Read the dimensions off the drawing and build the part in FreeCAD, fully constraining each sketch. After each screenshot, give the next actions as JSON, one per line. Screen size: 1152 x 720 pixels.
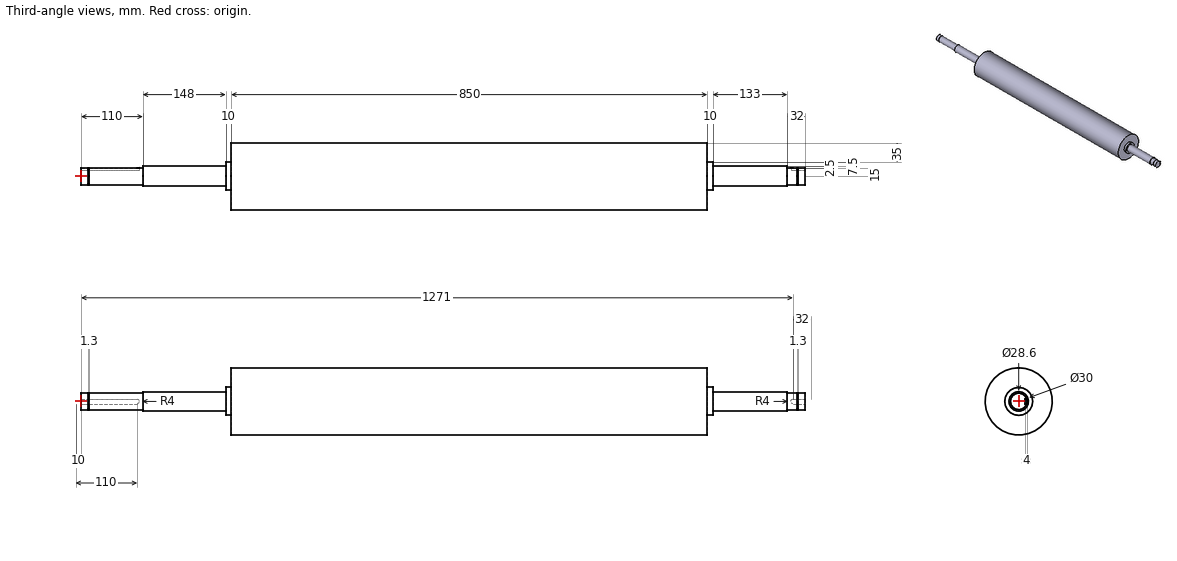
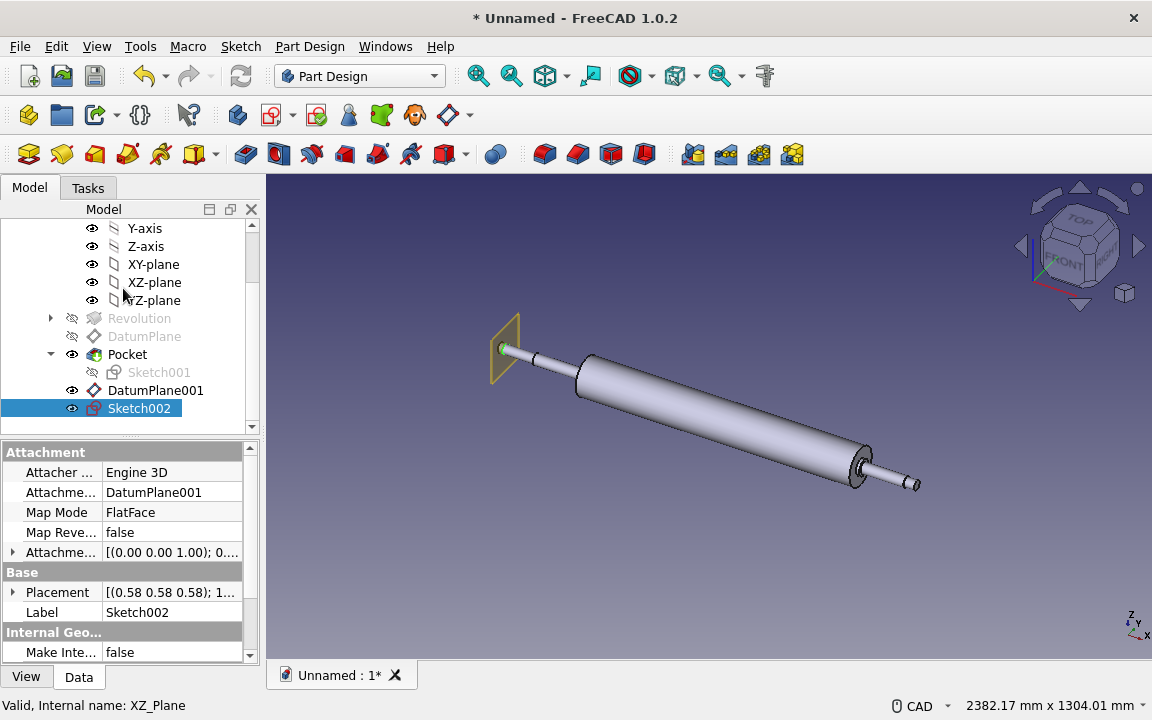
{"action": "left_click", "coordinate": [246, 154]}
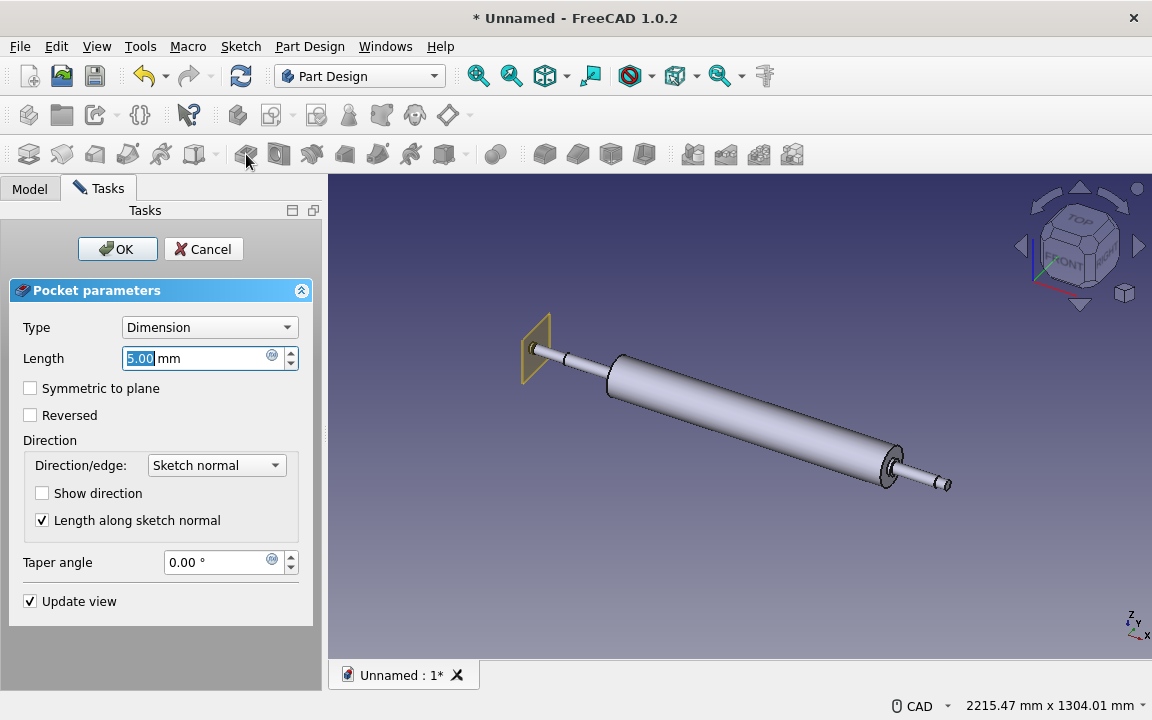
{"action": "type", "text": "1.3"}
{"action": "key", "text": "Tab"}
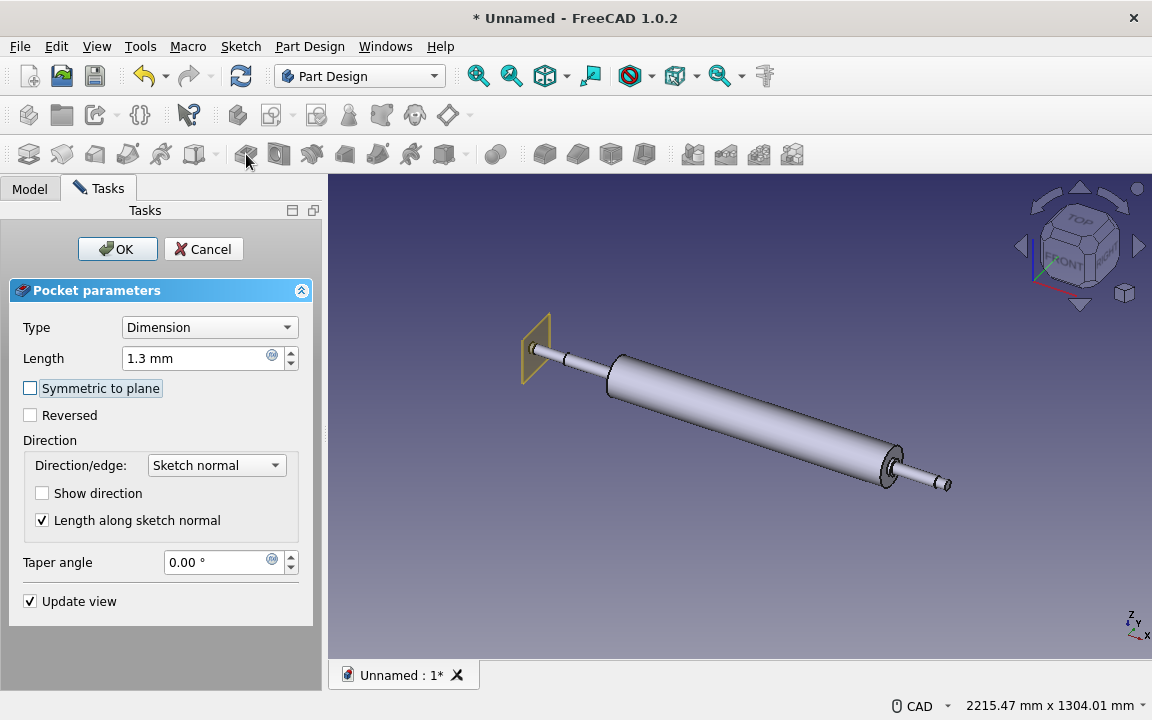
{"action": "left_click", "coordinate": [118, 249]}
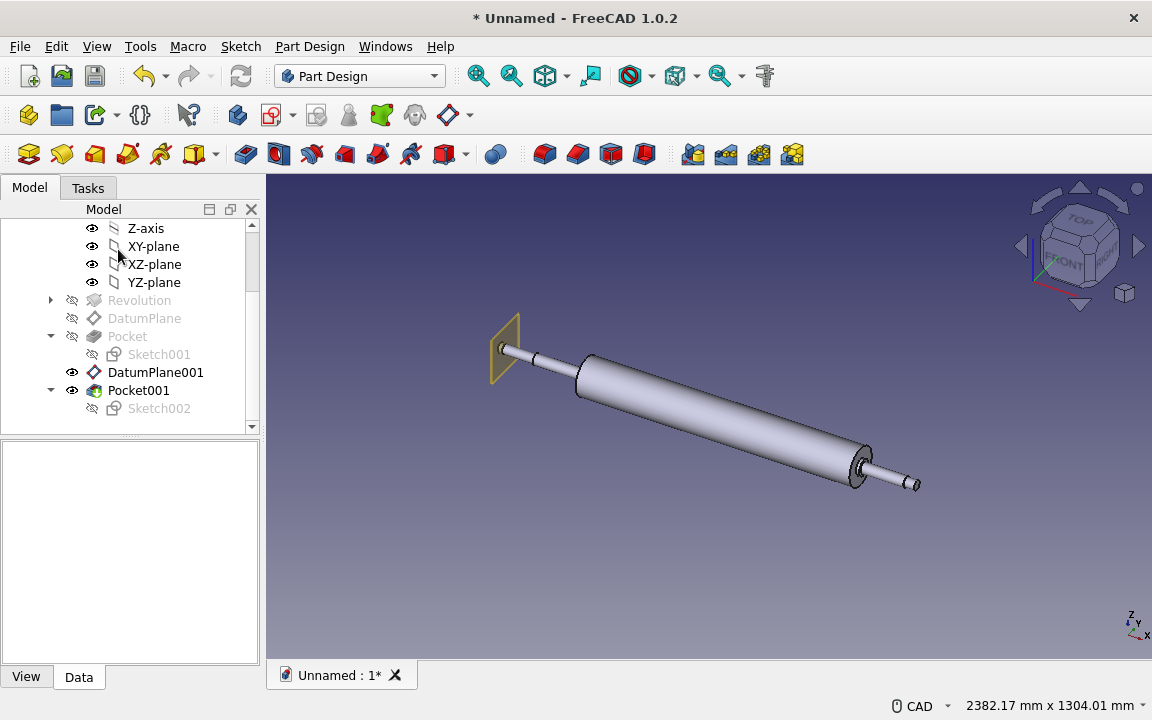
{"action": "left_click", "coordinate": [117, 372]}
{"action": "key", "text": "space"}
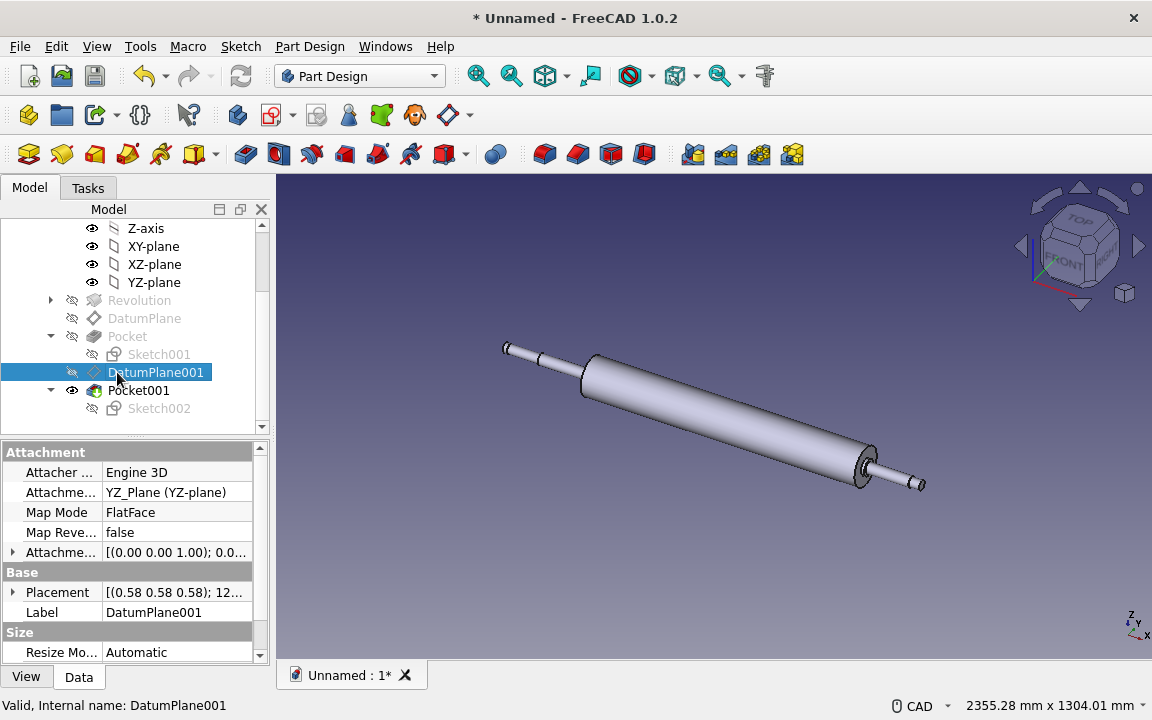
{"action": "scroll", "coordinate": [161, 314], "scroll_direction": "down", "scroll_amount": 3}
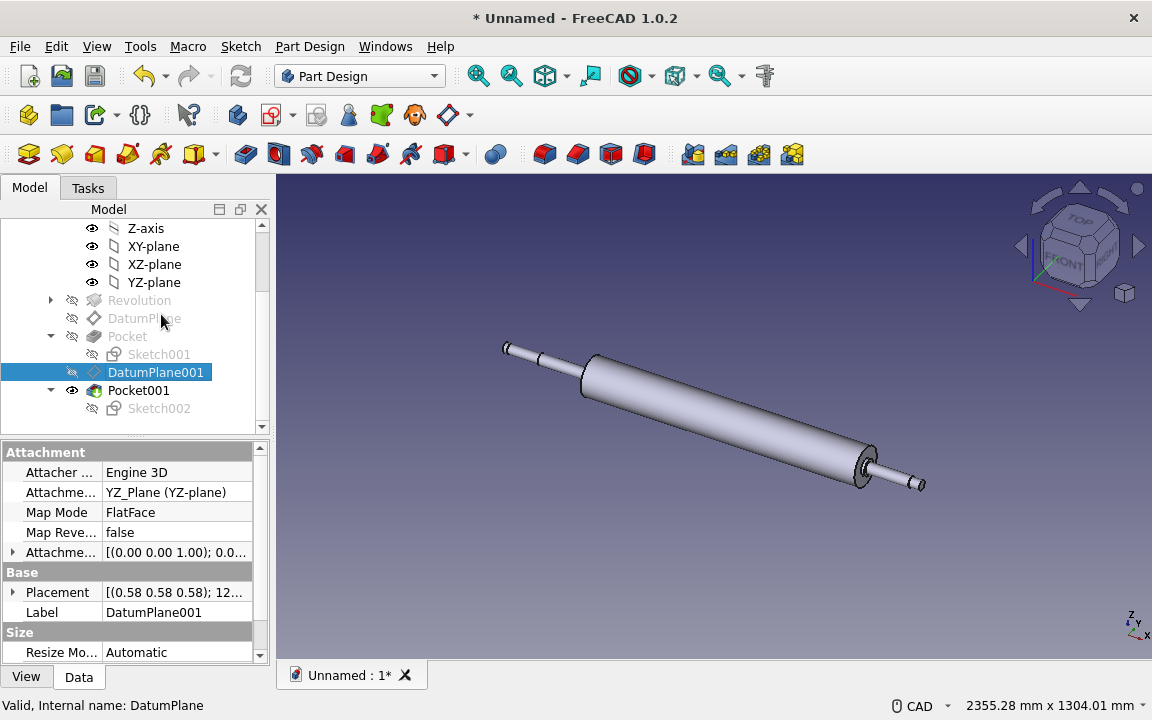
{"action": "scroll", "coordinate": [161, 314], "scroll_direction": "up", "scroll_amount": 15}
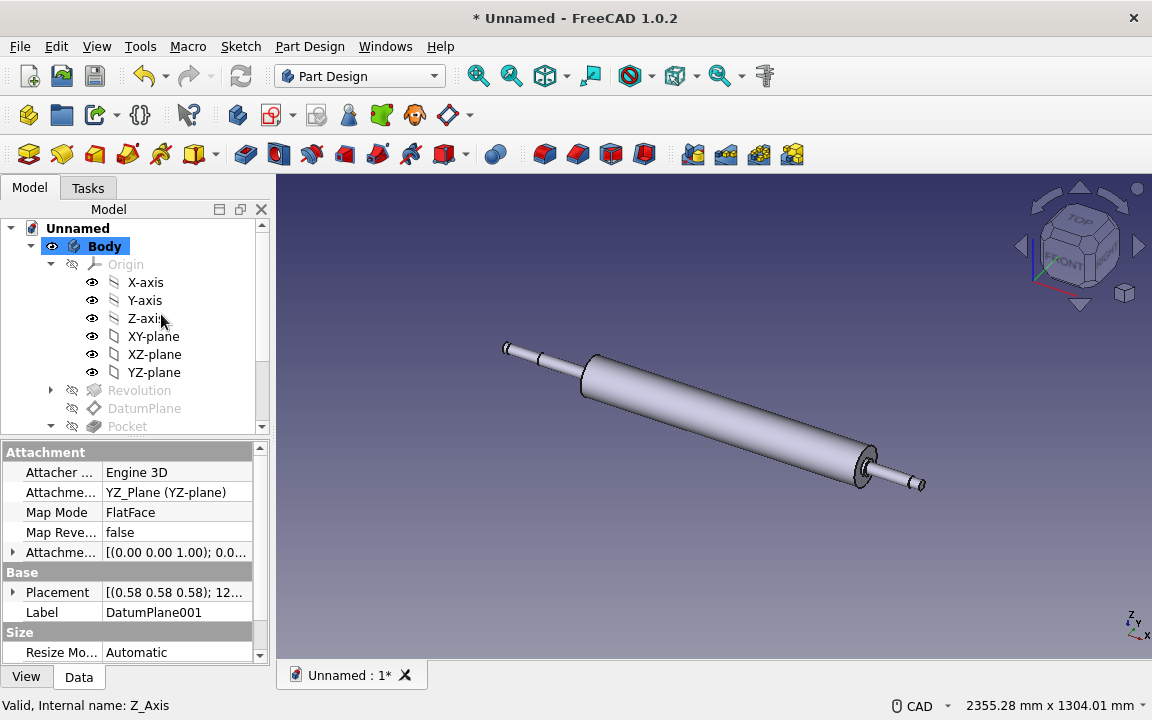
{"action": "left_click", "coordinate": [137, 354]}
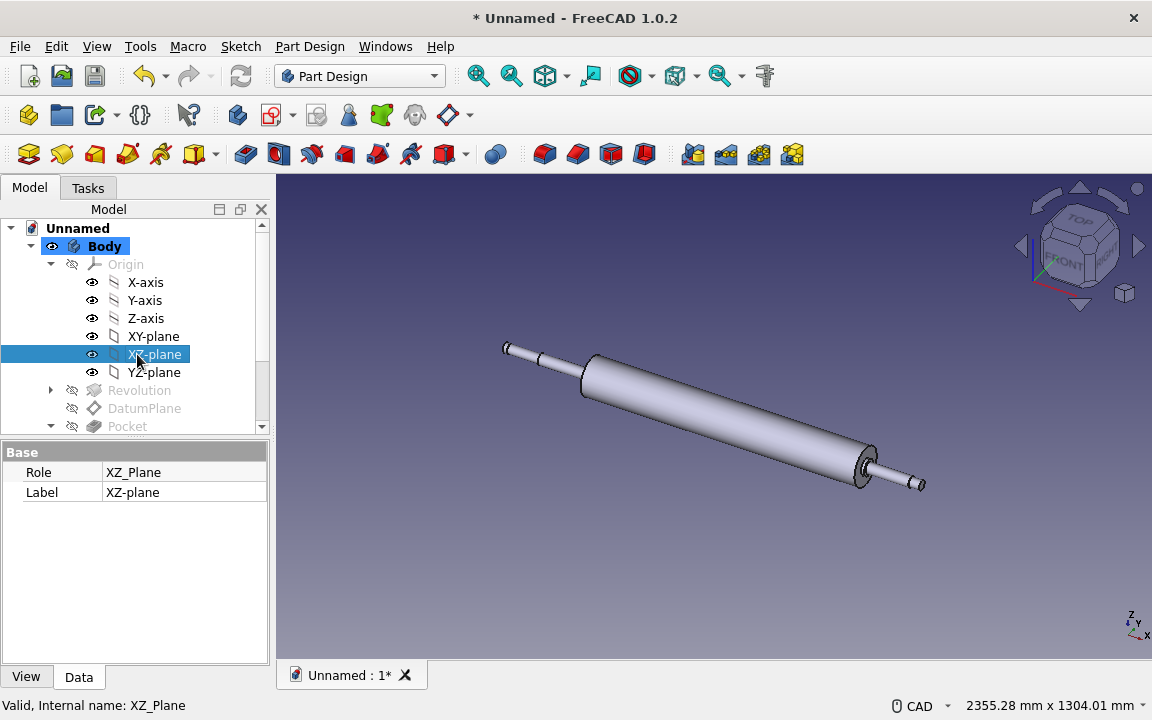
{"action": "left_click", "coordinate": [448, 116]}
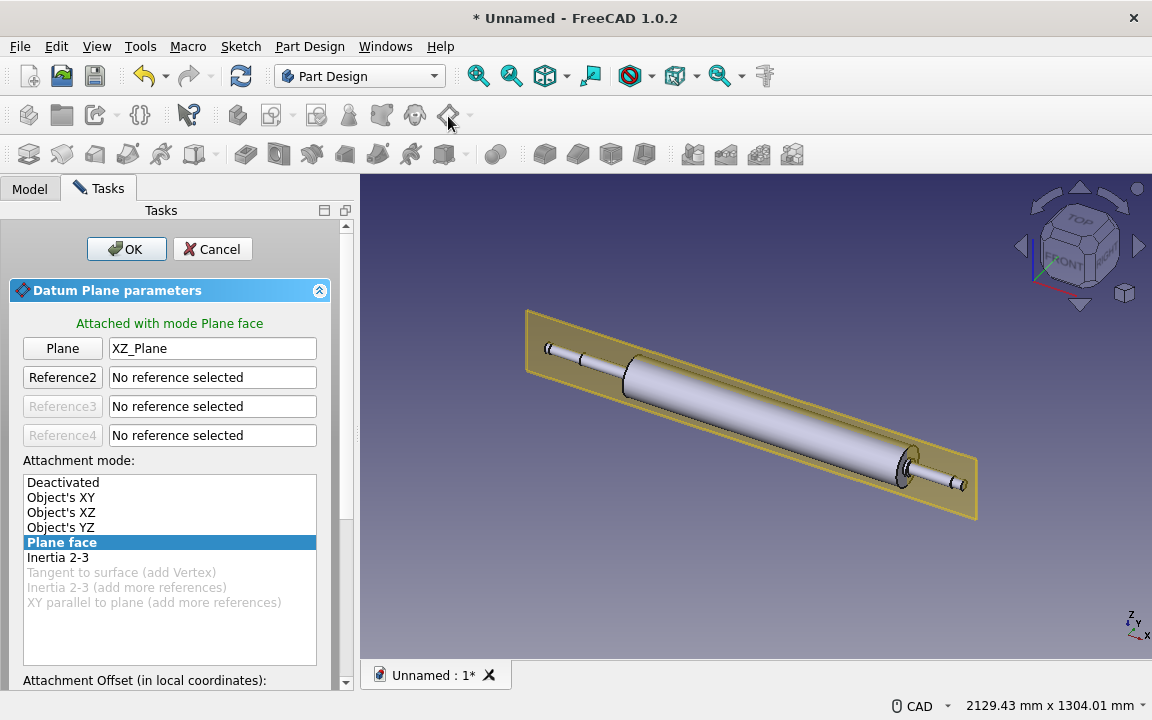
{"action": "scroll", "coordinate": [346, 455], "scroll_direction": "down", "scroll_amount": 3}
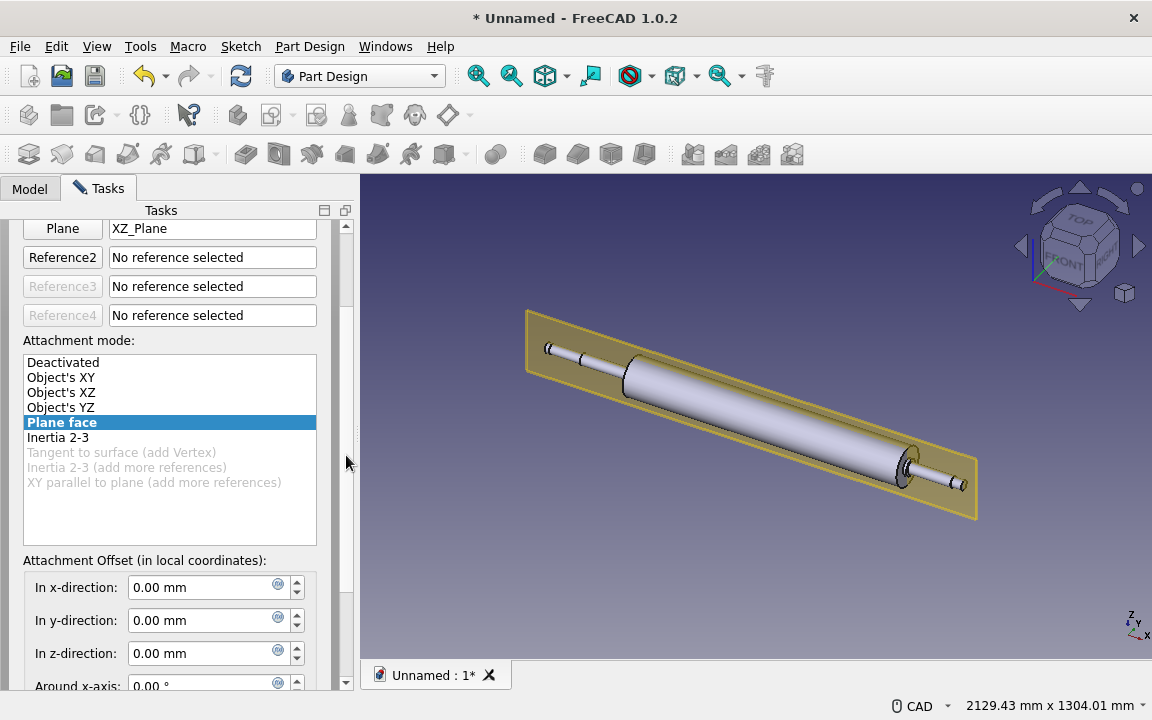
{"action": "triple_click", "coordinate": [210, 594]}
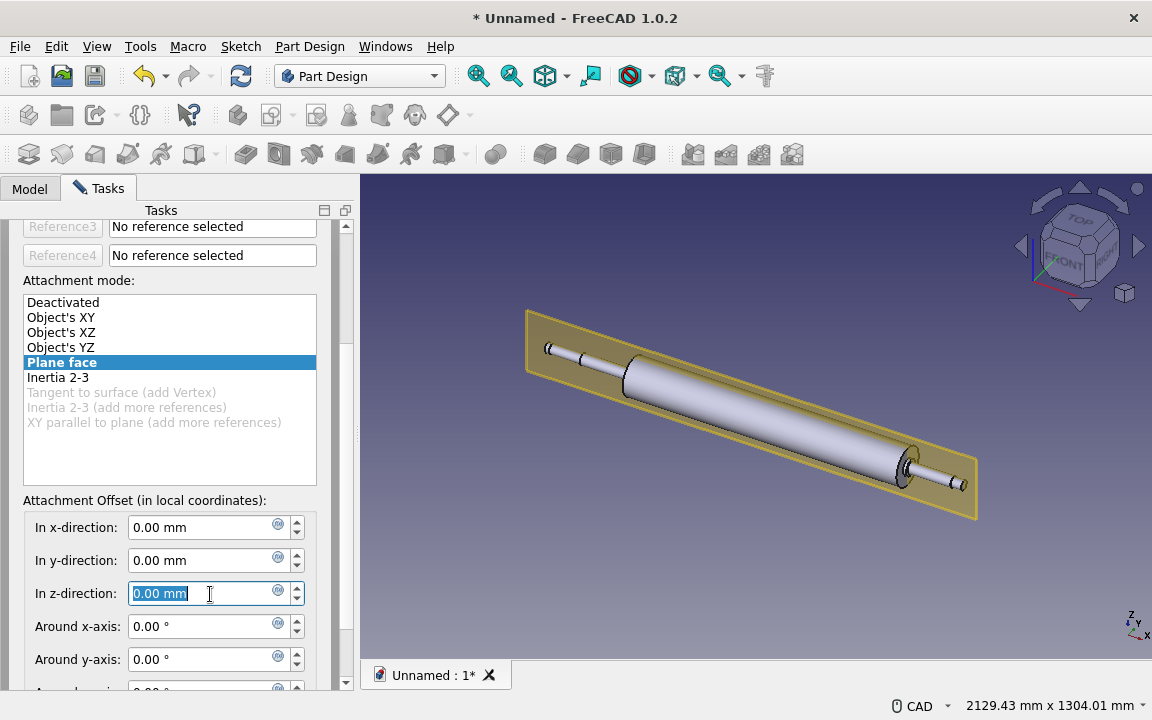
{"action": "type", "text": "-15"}
{"action": "key", "text": "Tab"}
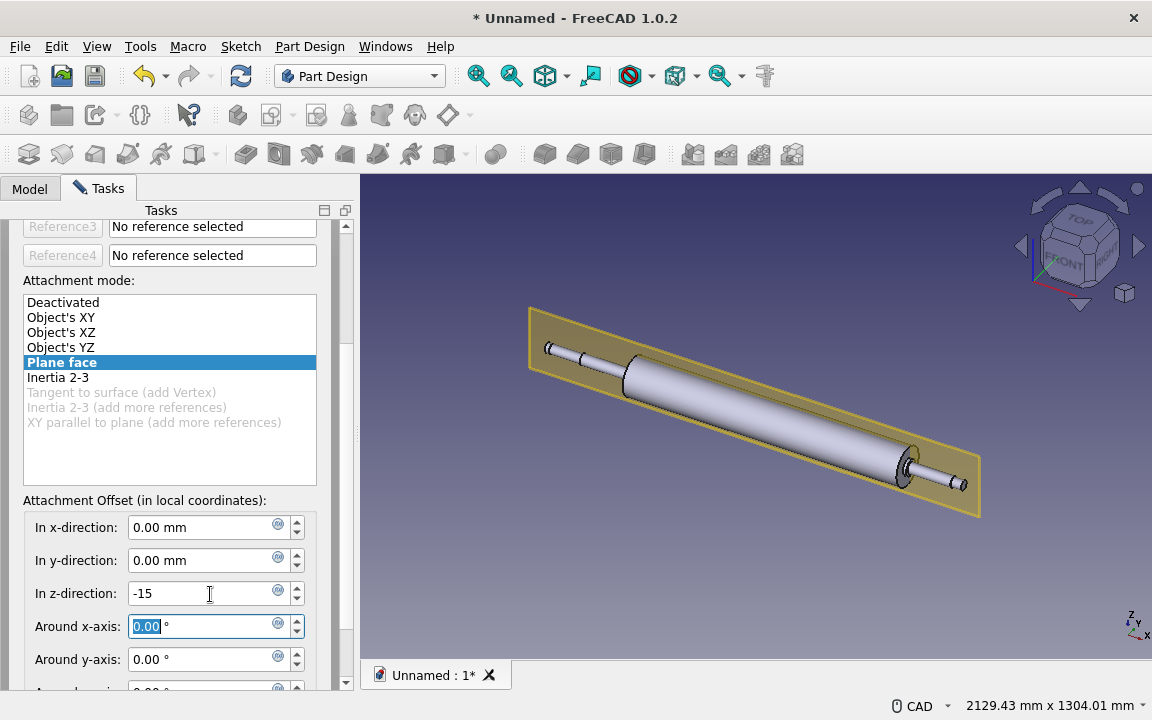
{"action": "scroll", "coordinate": [346, 455], "scroll_direction": "up", "scroll_amount": 4}